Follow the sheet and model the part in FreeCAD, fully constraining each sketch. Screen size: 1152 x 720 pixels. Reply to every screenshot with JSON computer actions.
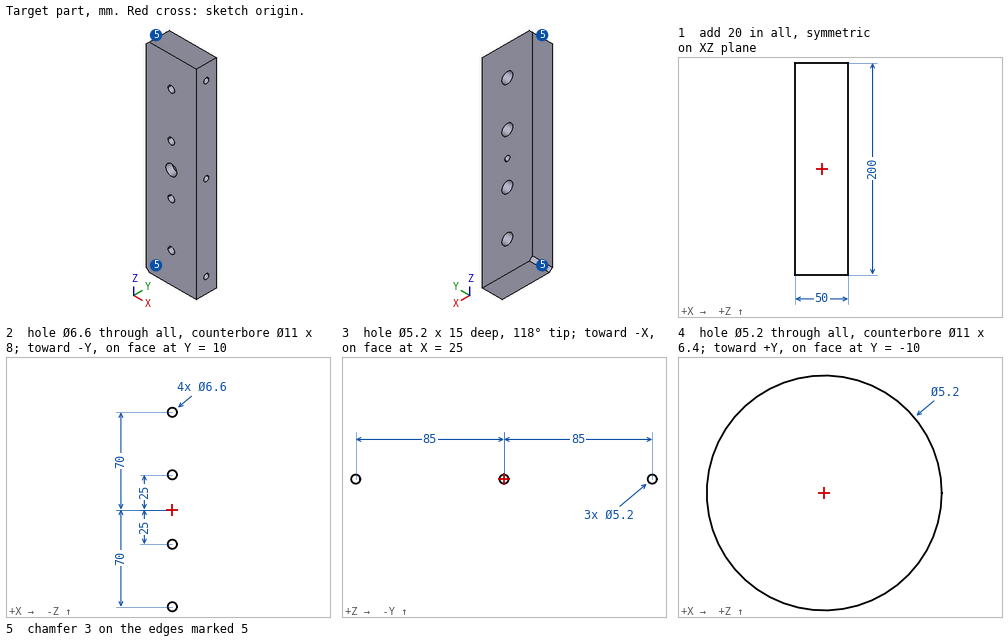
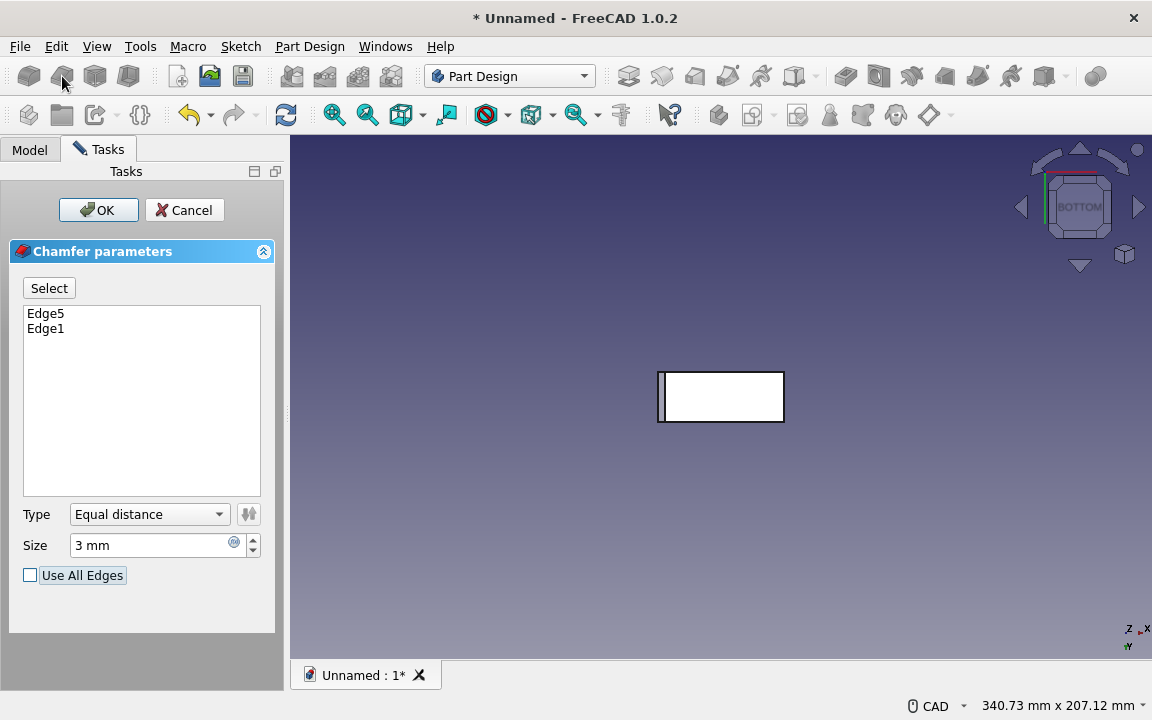
{"action": "left_click", "coordinate": [99, 210]}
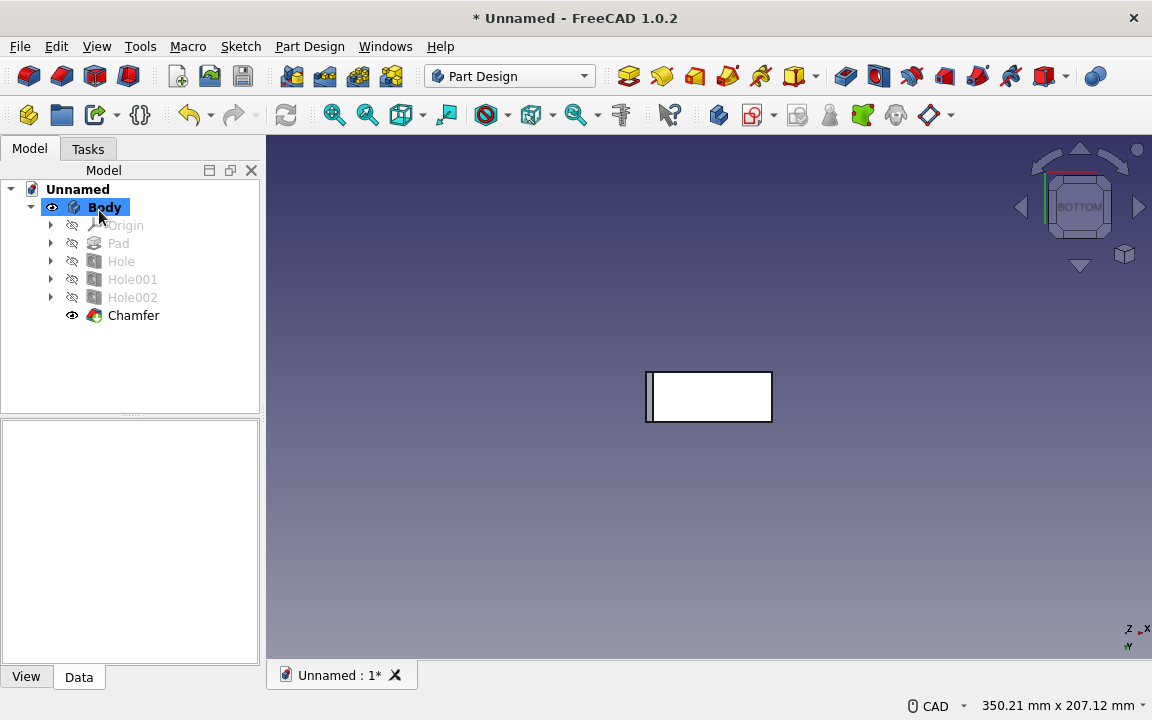
{"action": "key", "text": "0"}